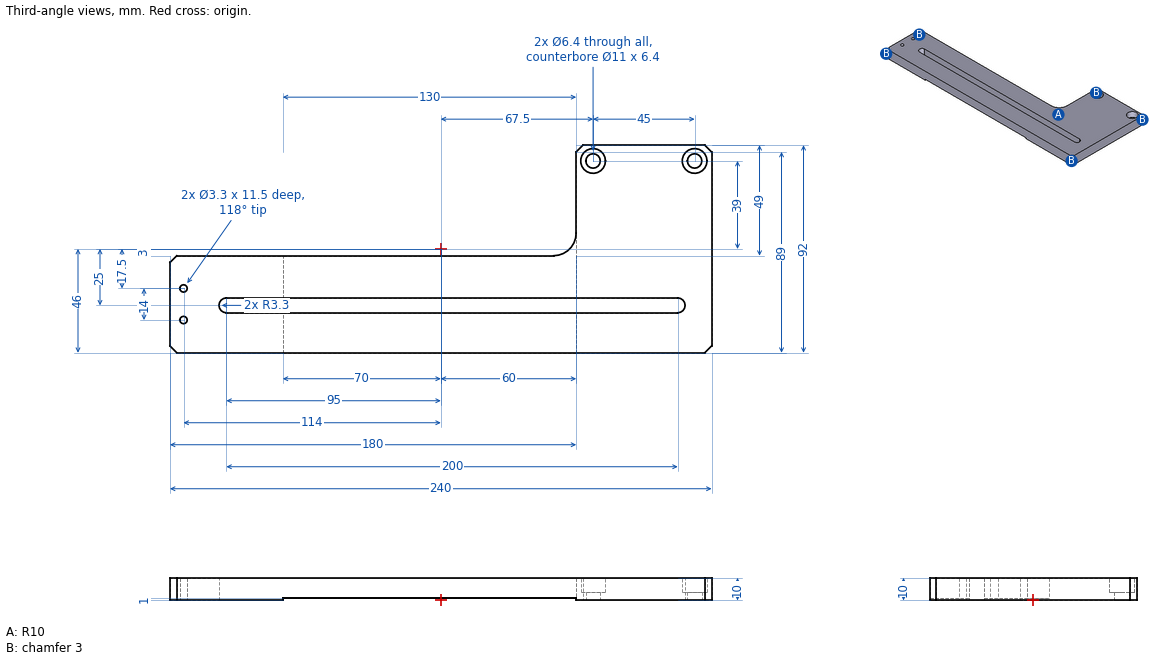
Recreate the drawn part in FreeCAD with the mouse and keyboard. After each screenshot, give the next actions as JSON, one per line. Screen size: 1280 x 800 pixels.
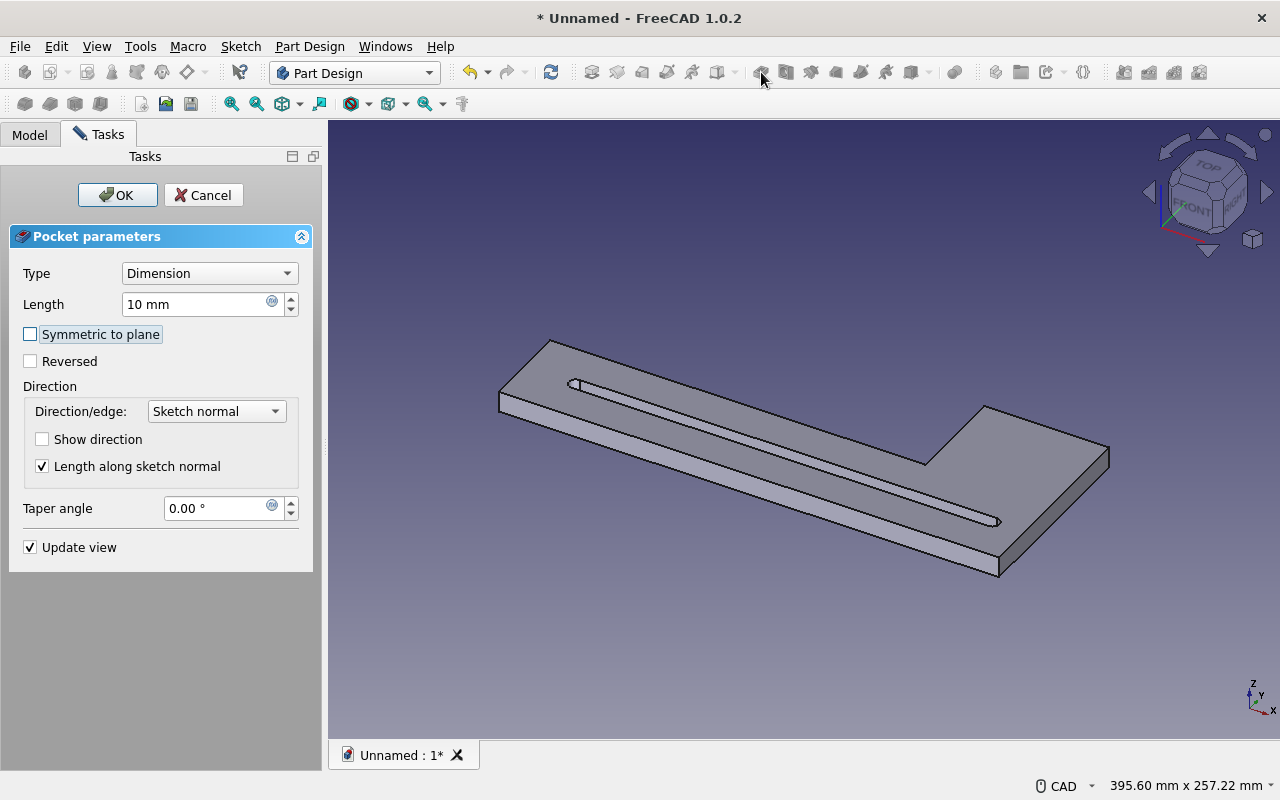
{"action": "left_click", "coordinate": [118, 195]}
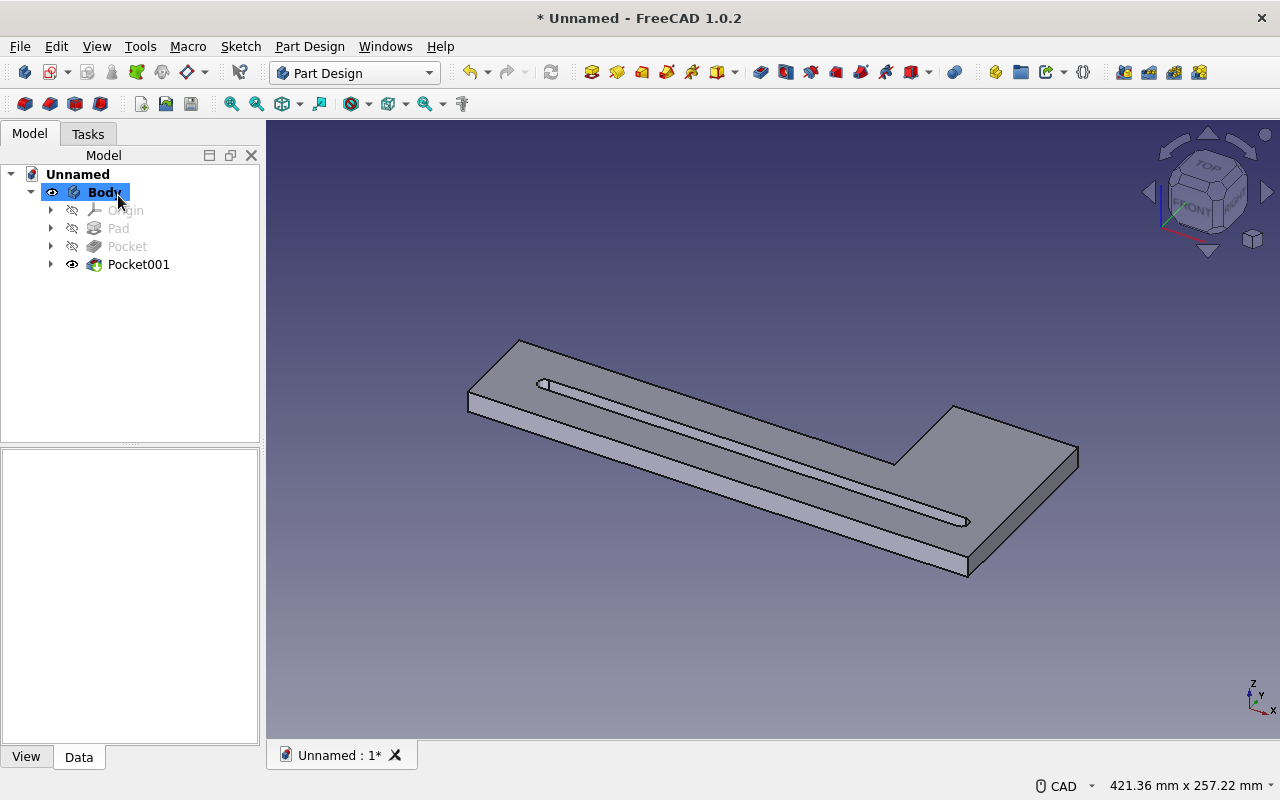
{"action": "key", "text": "0"}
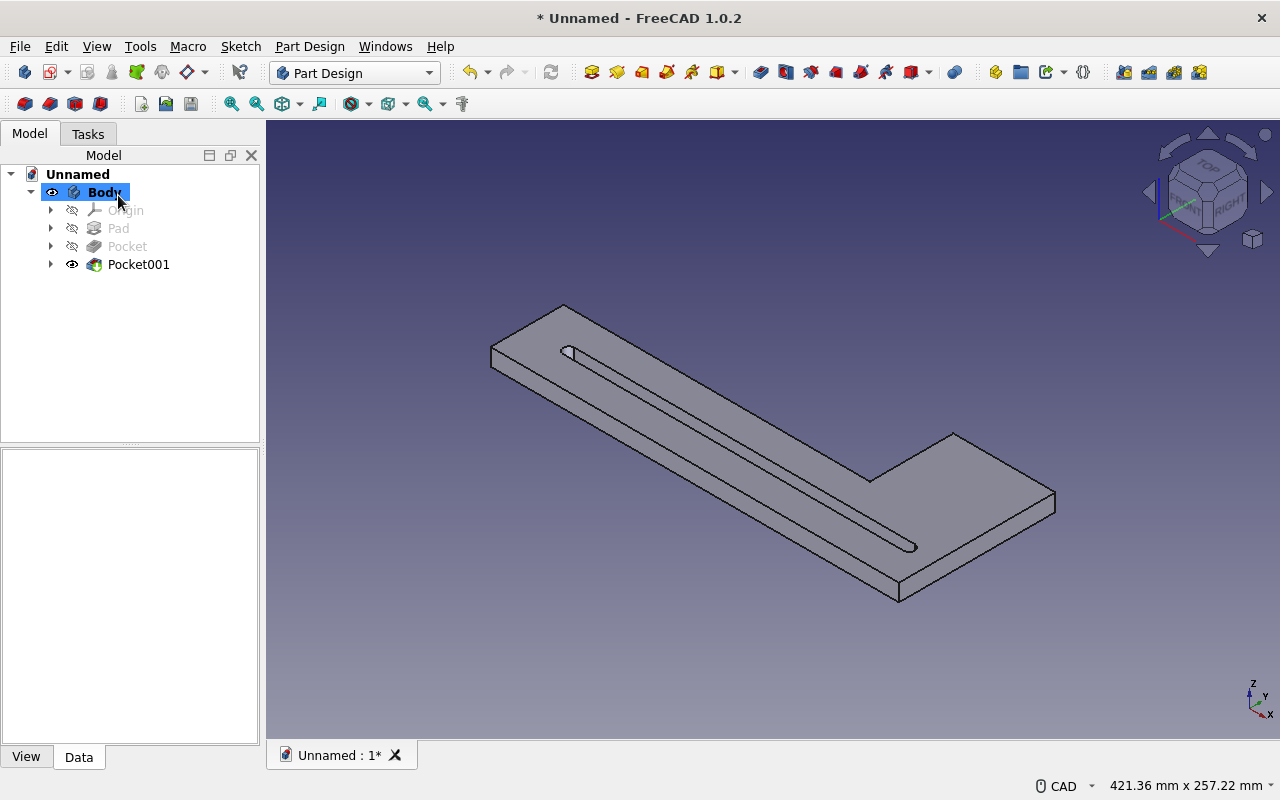
{"action": "key", "text": "2"}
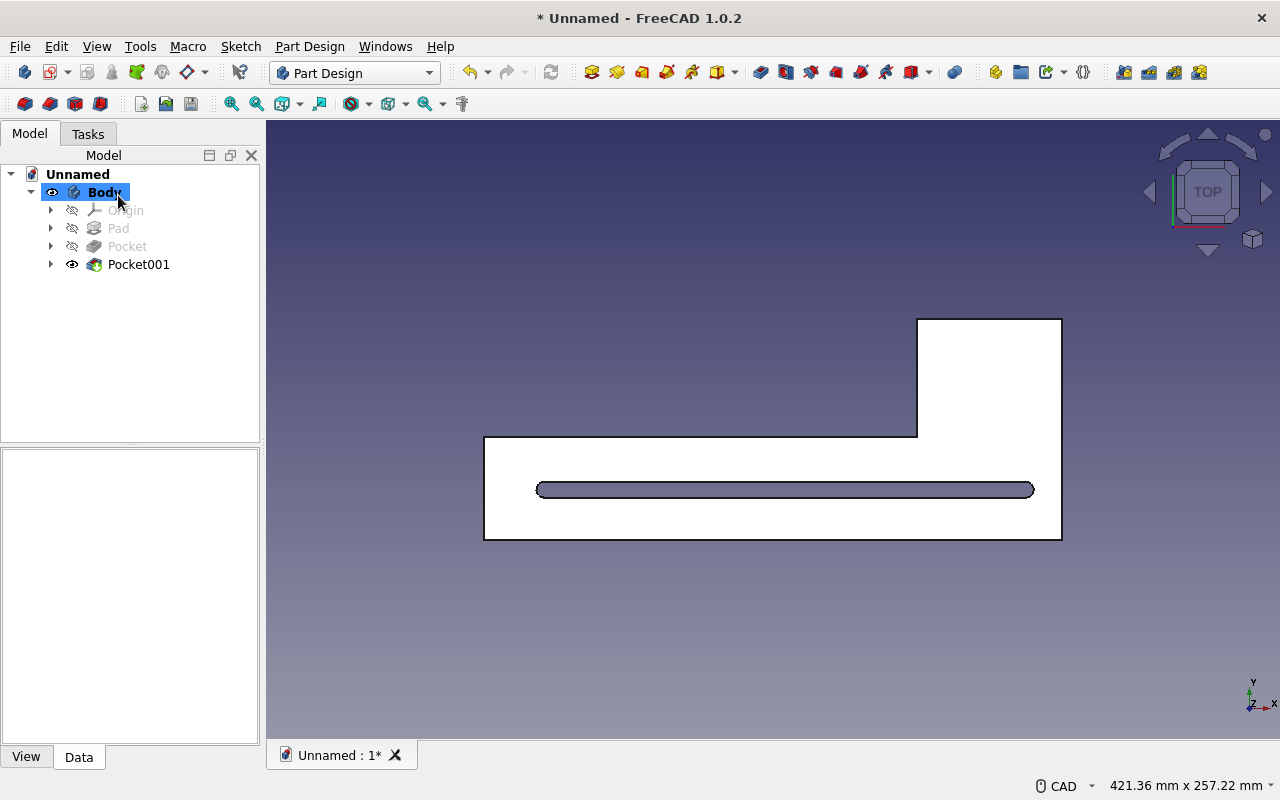
{"action": "key", "text": "1"}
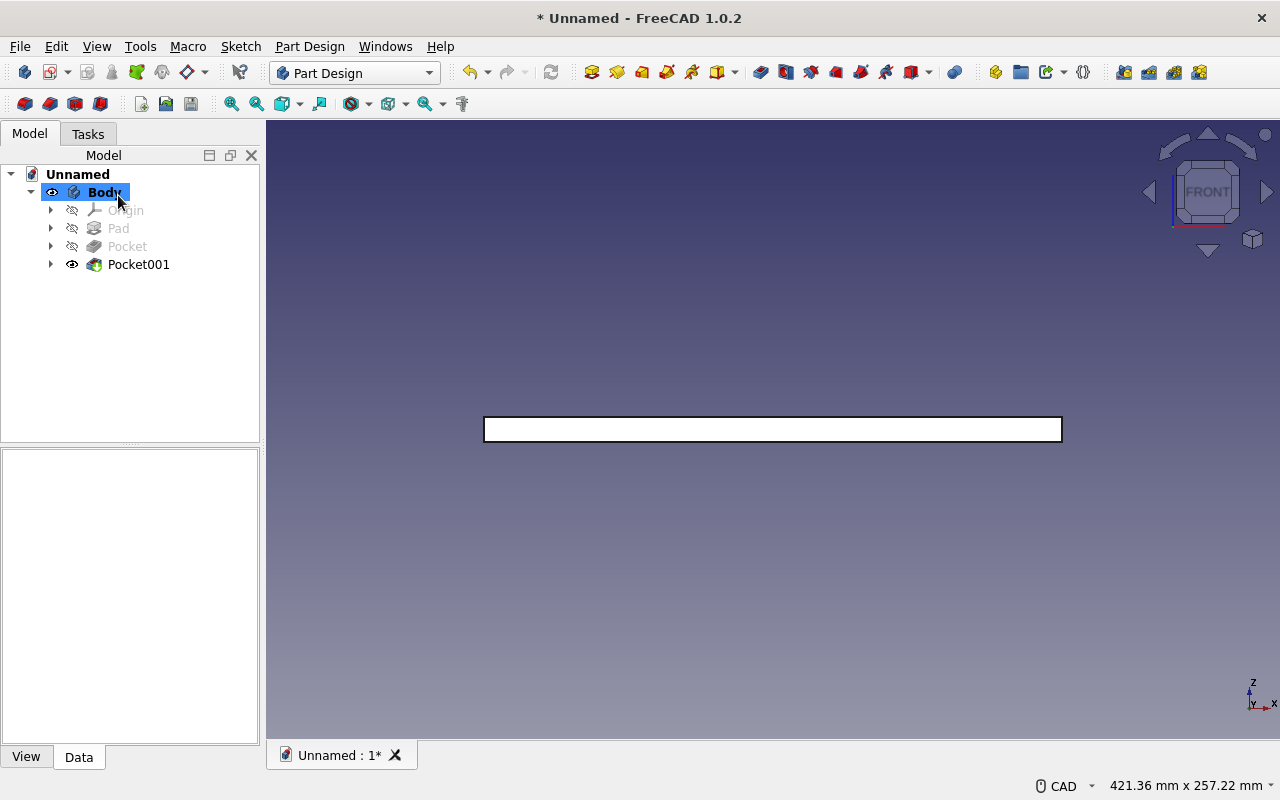
{"action": "key", "text": "3"}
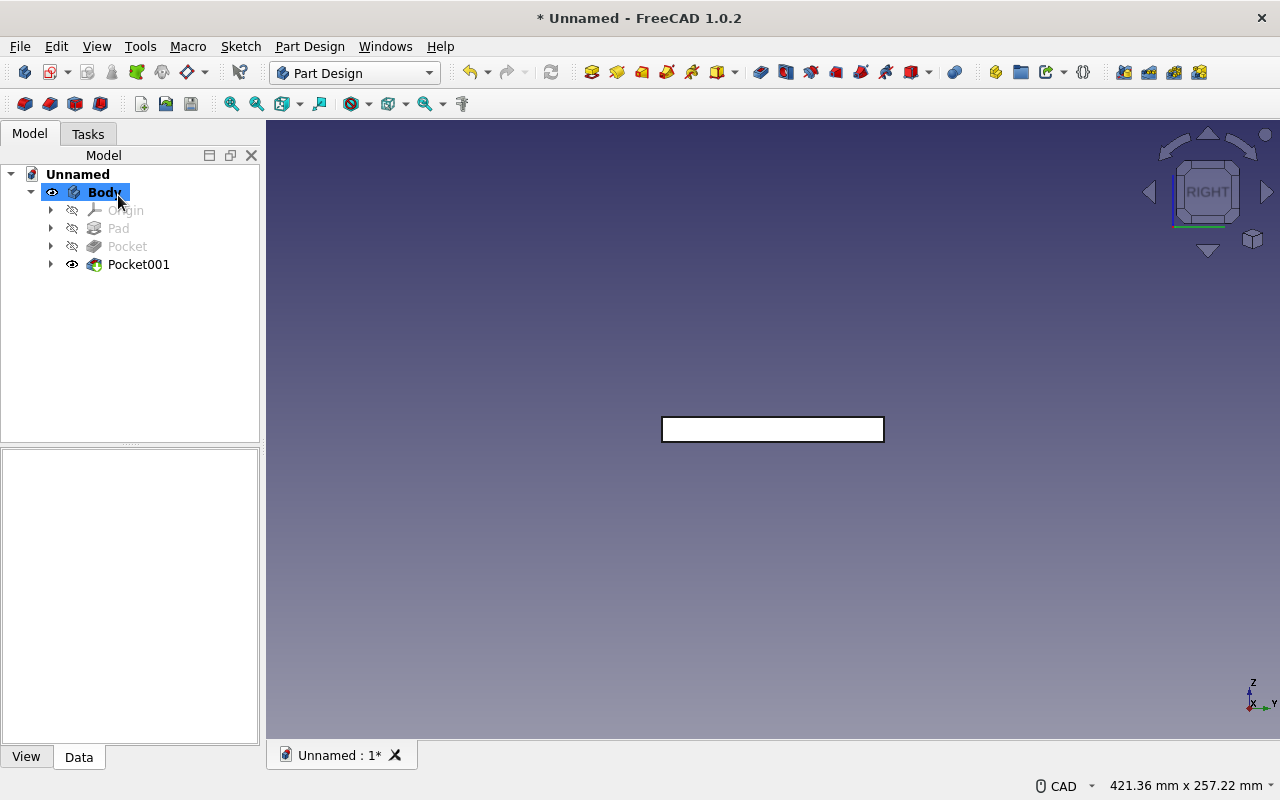
{"action": "key", "text": "v f"}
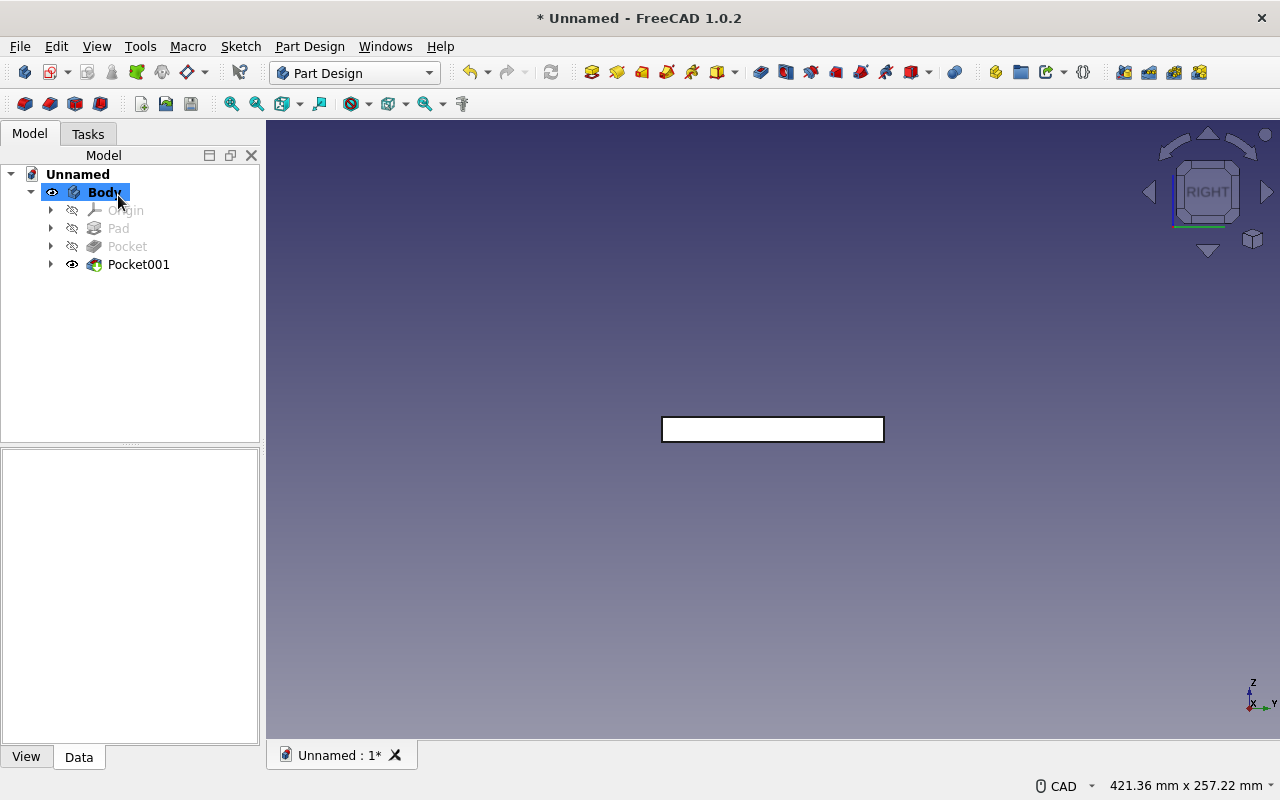
{"action": "key", "text": "5"}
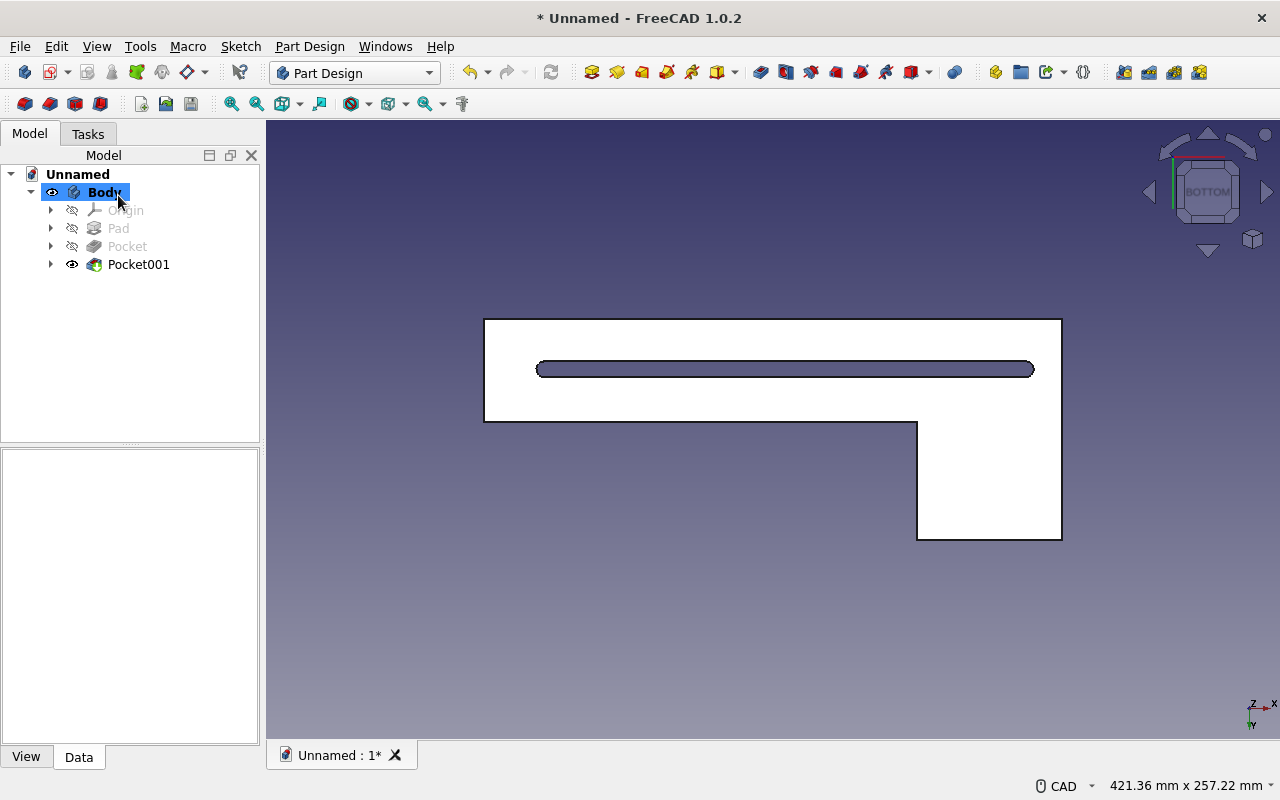
{"action": "key", "text": "4"}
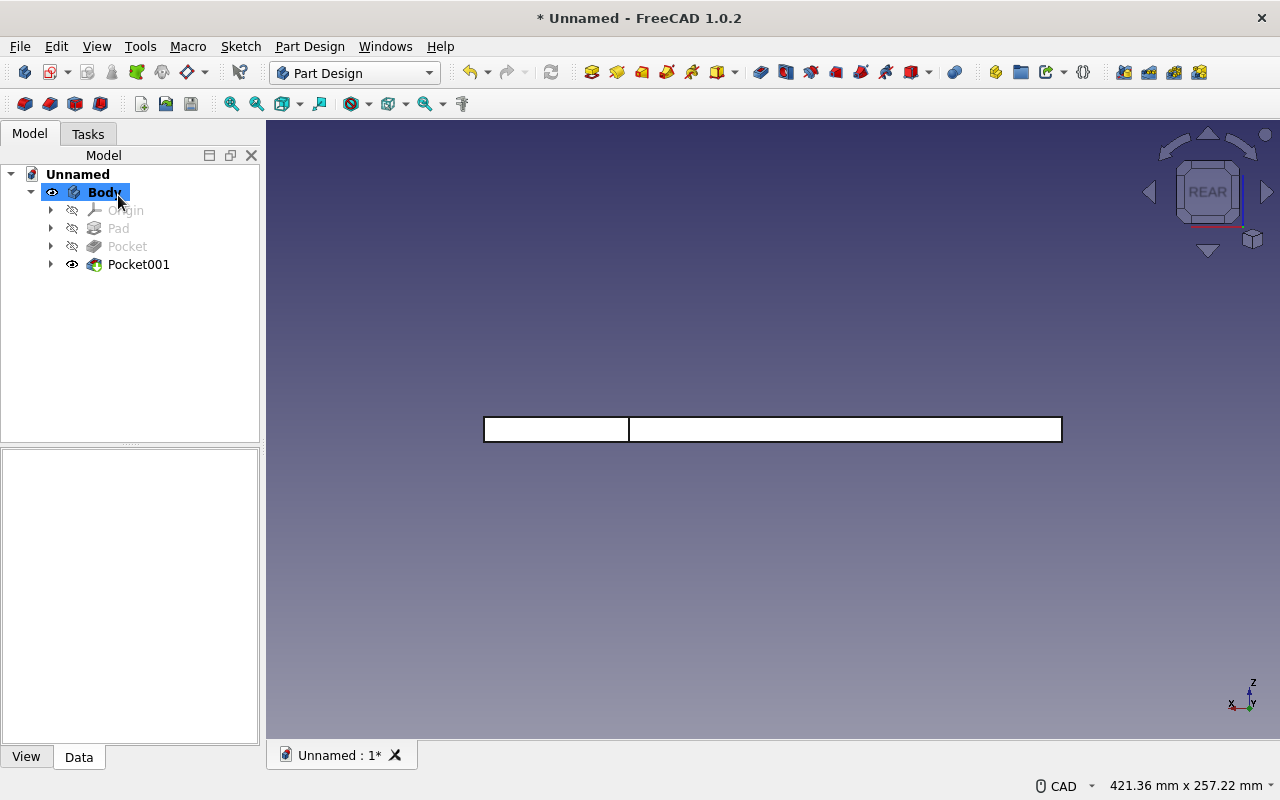
{"action": "key", "text": "6"}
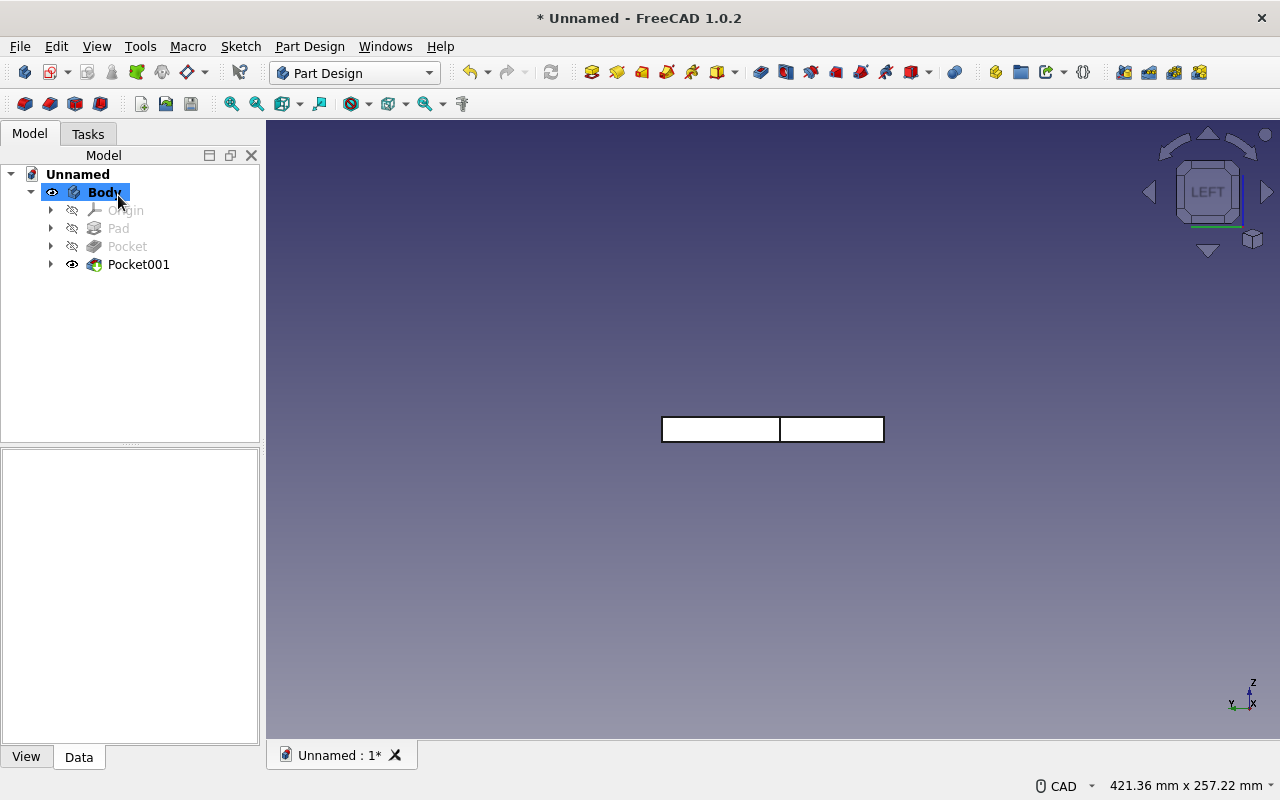
{"action": "left_click", "coordinate": [232, 104]}